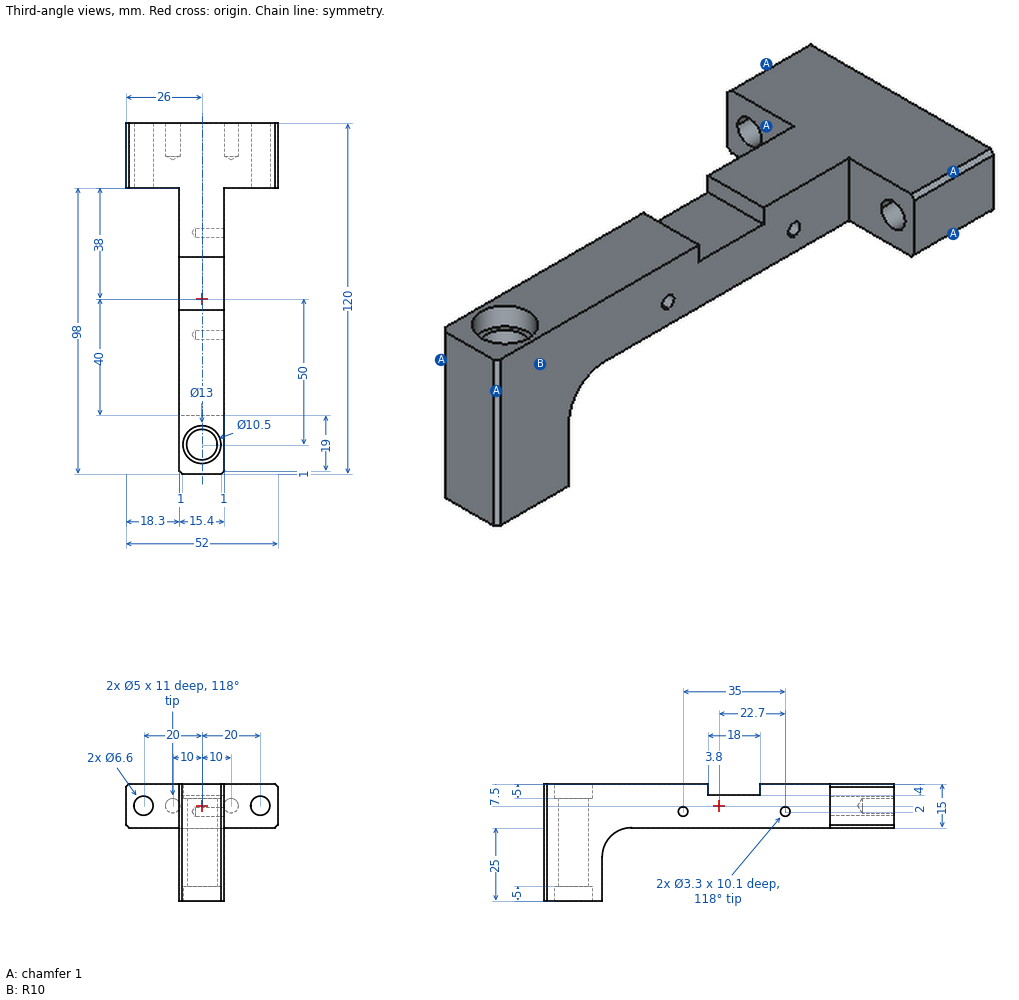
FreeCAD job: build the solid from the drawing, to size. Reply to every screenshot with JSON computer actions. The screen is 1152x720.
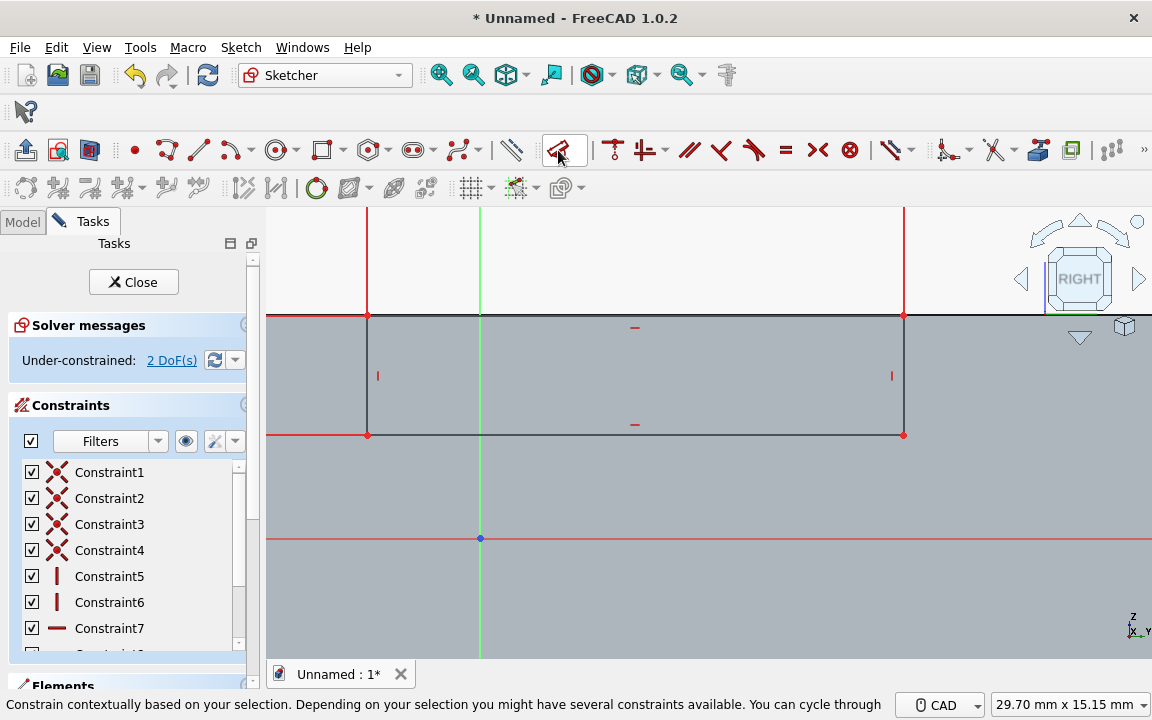
{"action": "left_click", "coordinate": [367, 316]}
{"action": "left_click", "coordinate": [424, 573]}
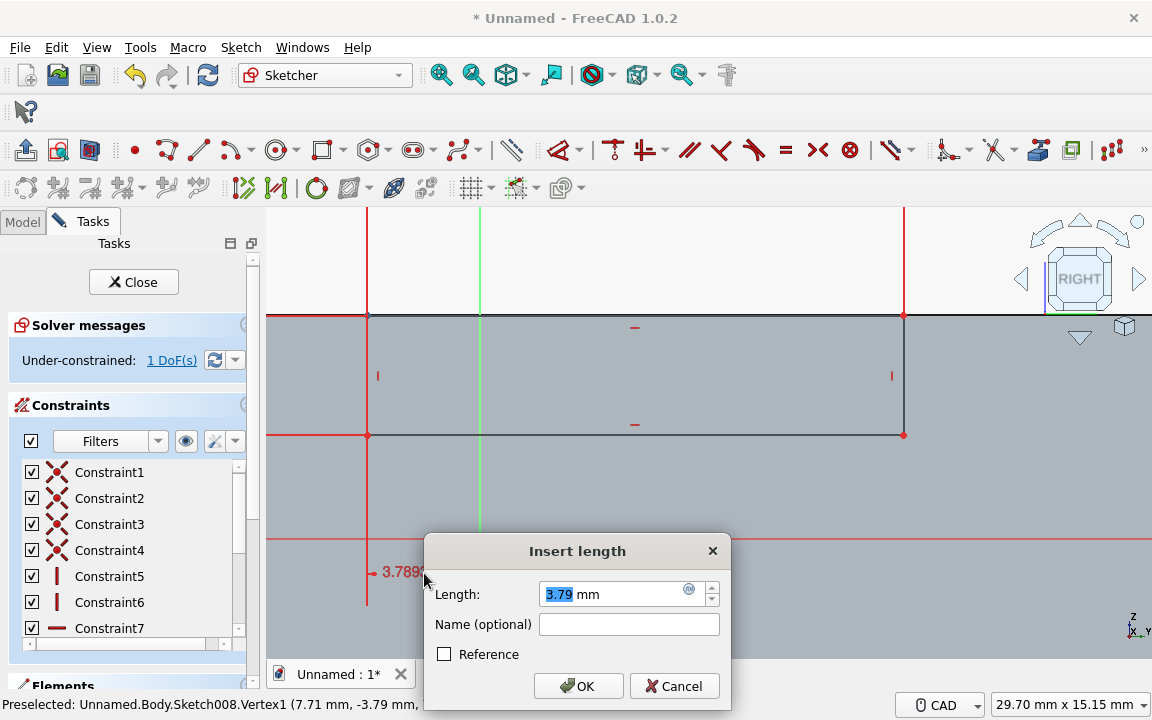
{"action": "type", "text": "3.8"}
{"action": "key", "text": "Return"}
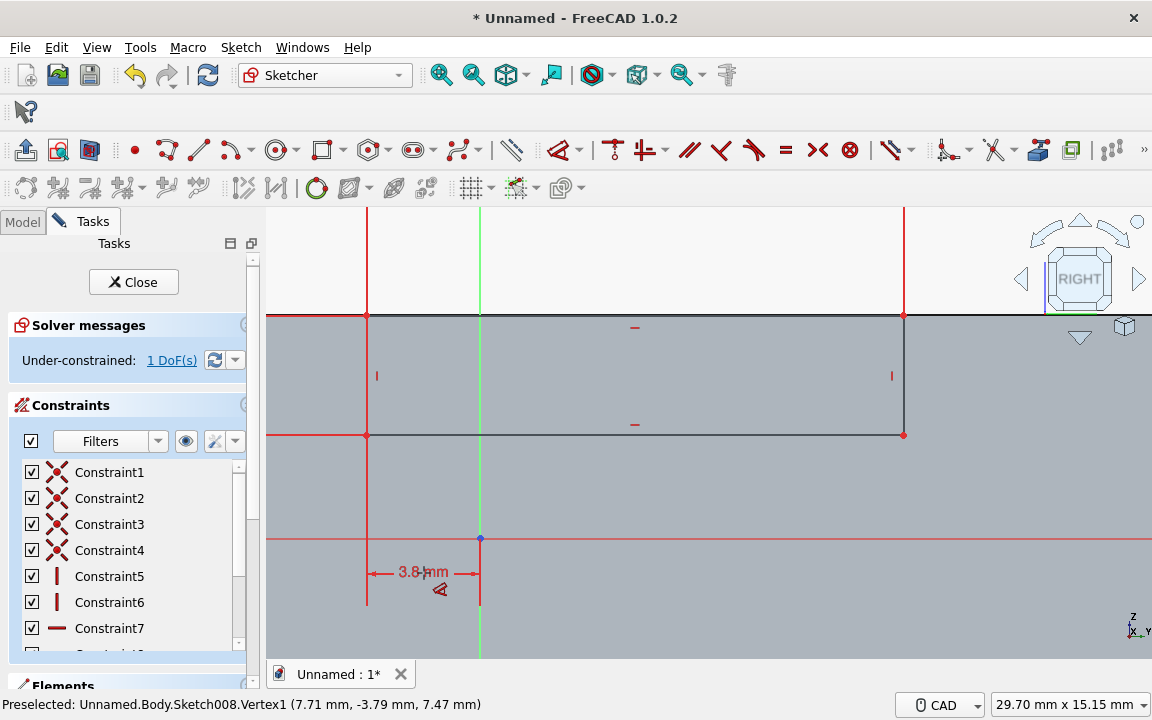
{"action": "left_click", "coordinate": [367, 316]}
{"action": "left_click", "coordinate": [333, 427]}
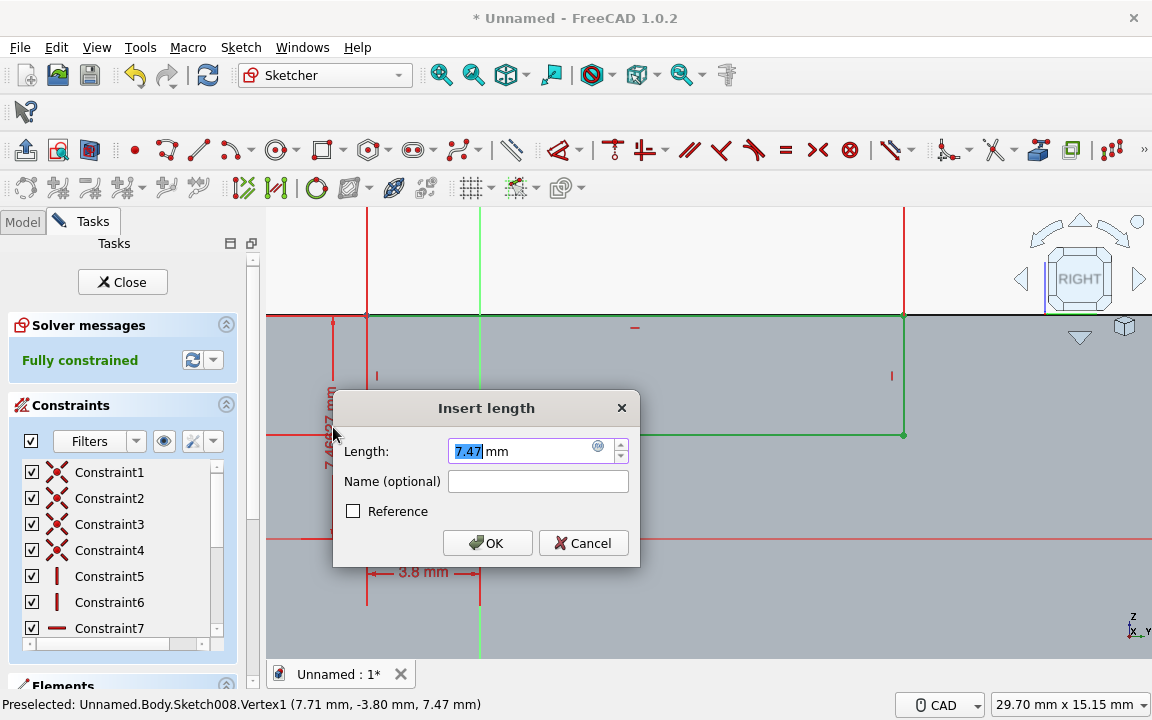
{"action": "type", "text": "7.5"}
{"action": "key", "text": "Return"}
{"action": "key", "text": "Escape"}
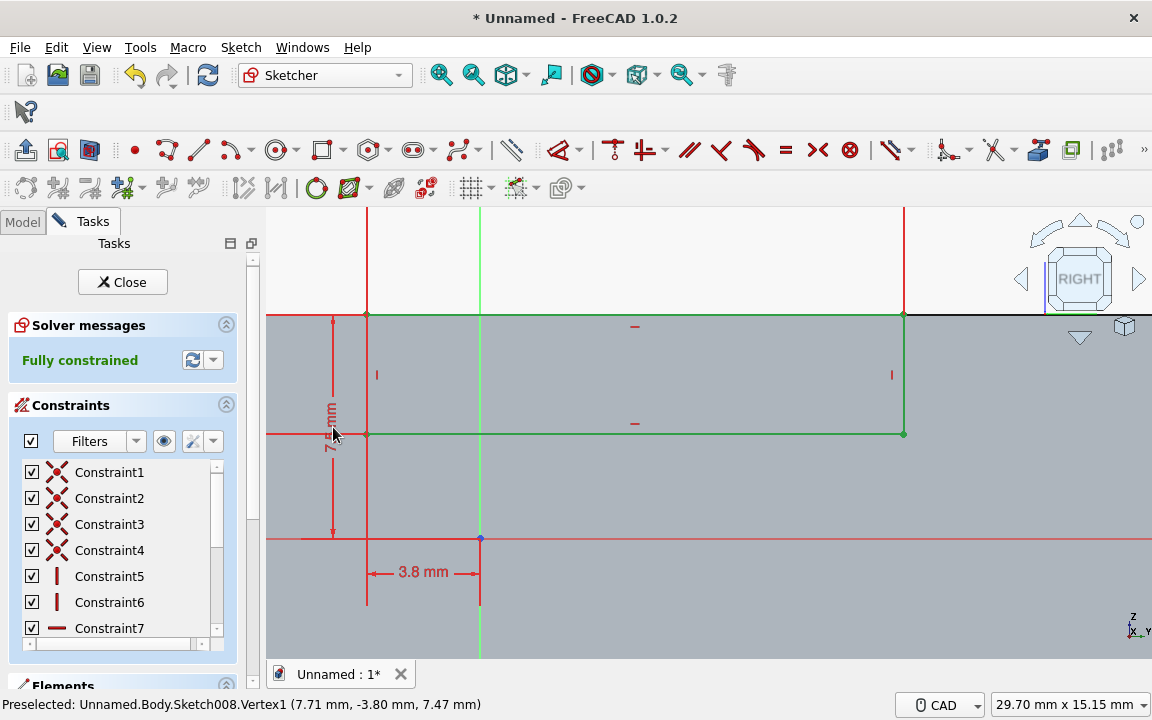
{"action": "left_click", "coordinate": [123, 282]}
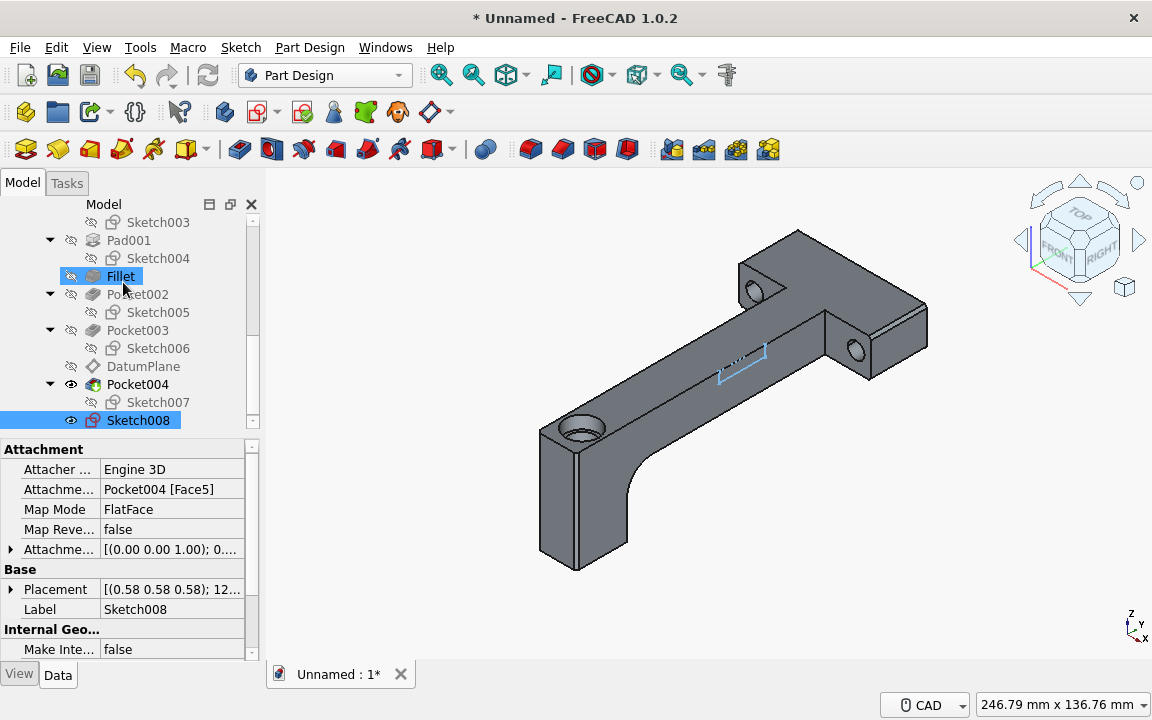
{"action": "left_click", "coordinate": [240, 150]}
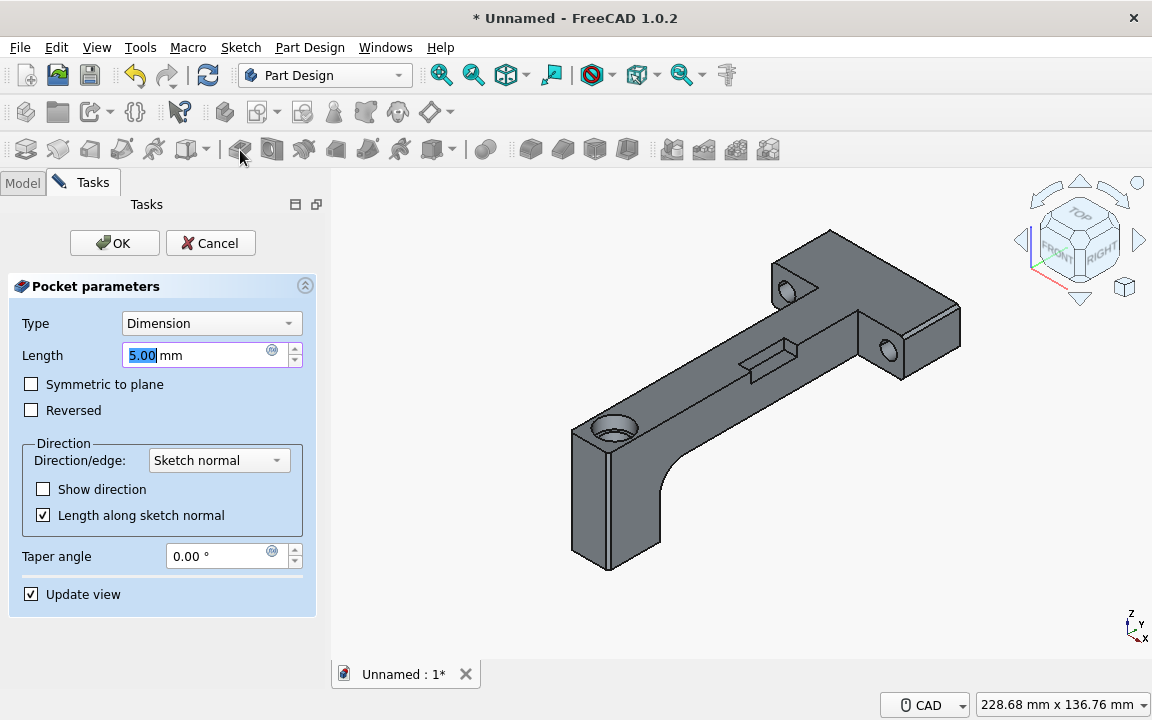
{"action": "left_click", "coordinate": [212, 324]}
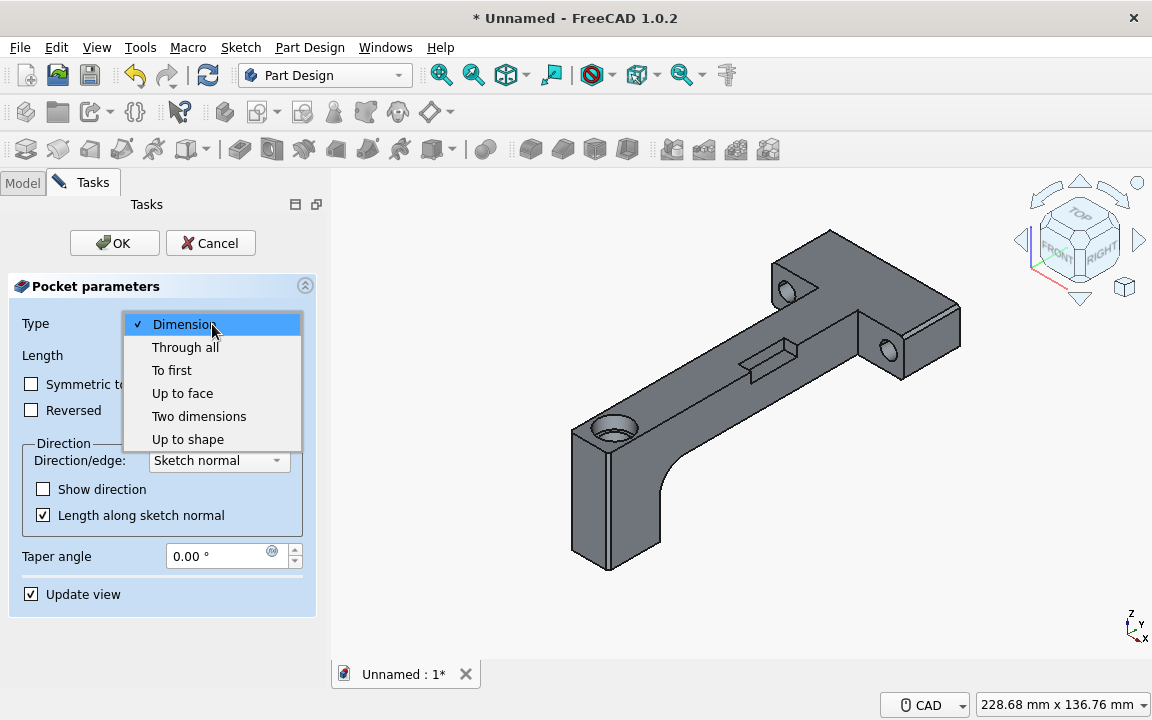
{"action": "left_click", "coordinate": [212, 348]}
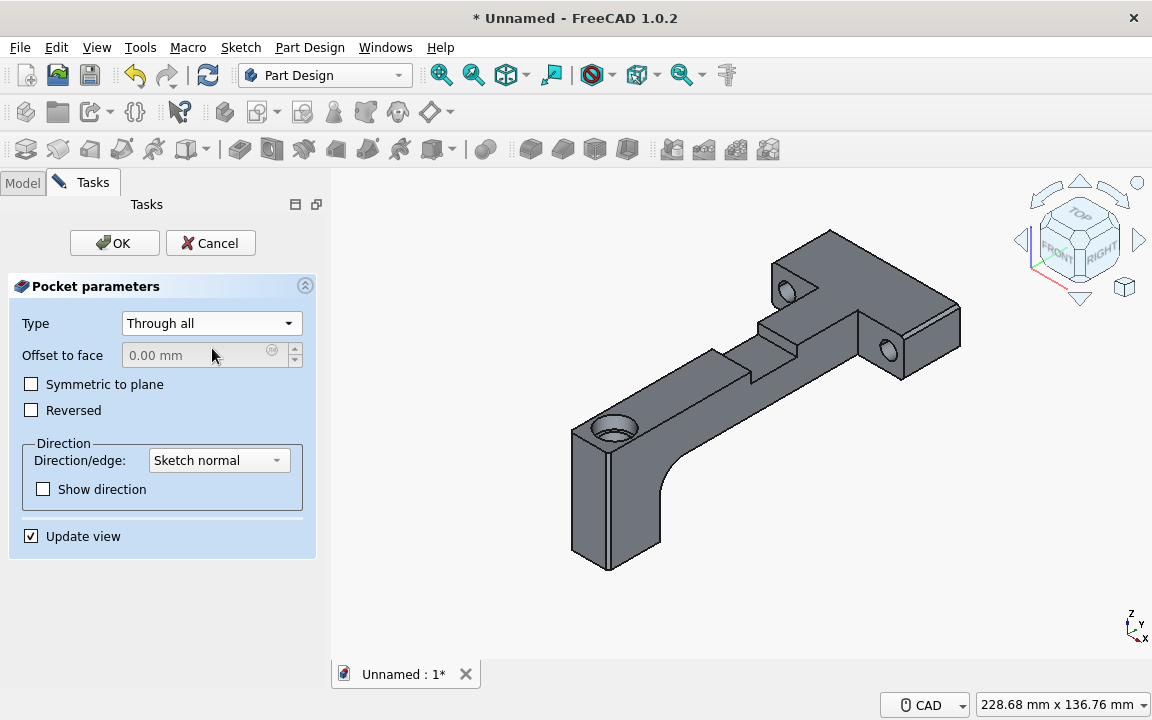
{"action": "left_click", "coordinate": [115, 243]}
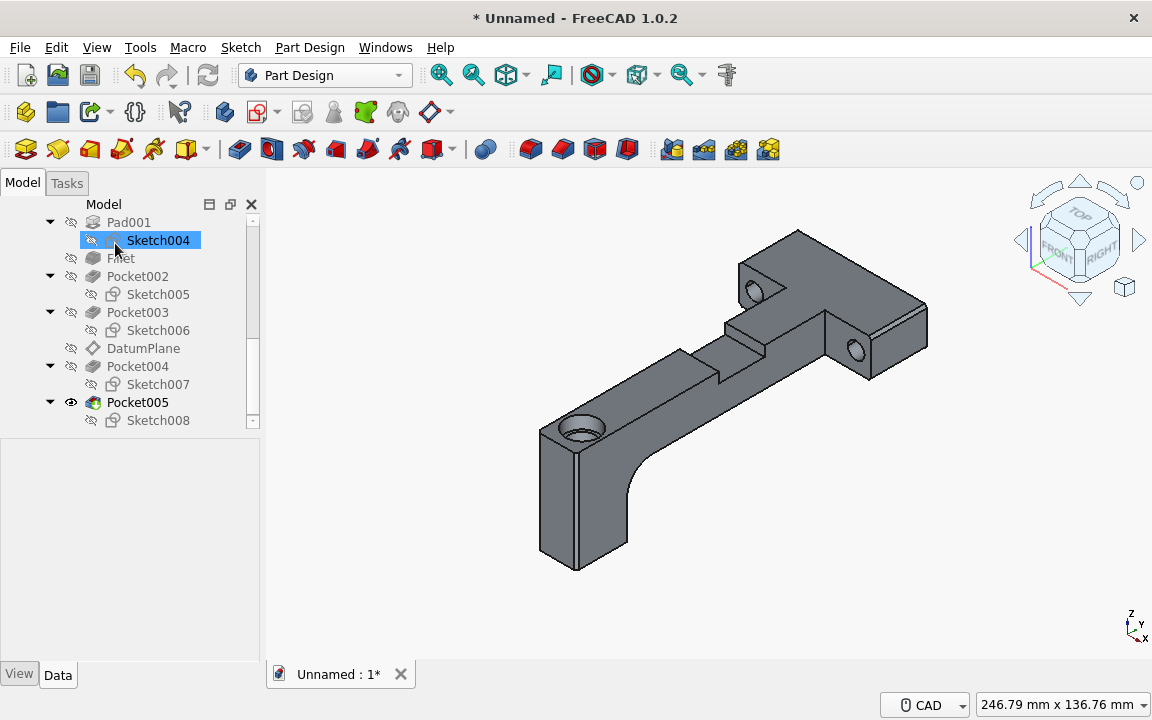
{"action": "left_click", "coordinate": [632, 446]}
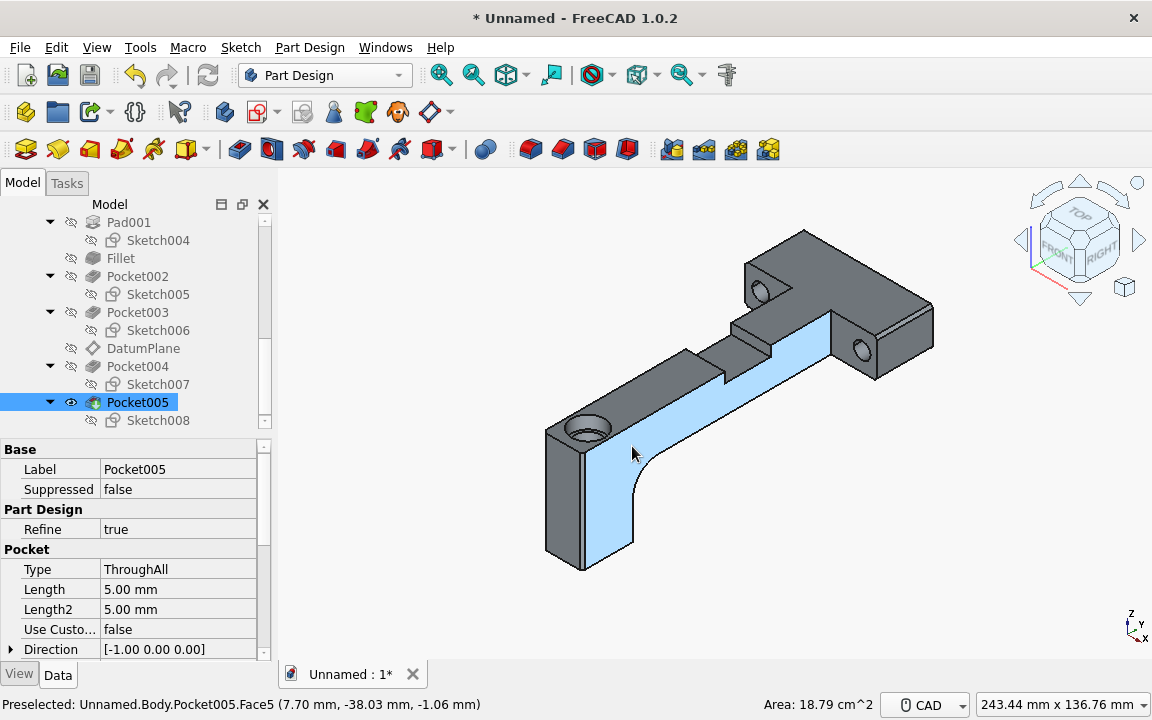
{"action": "left_click", "coordinate": [258, 112]}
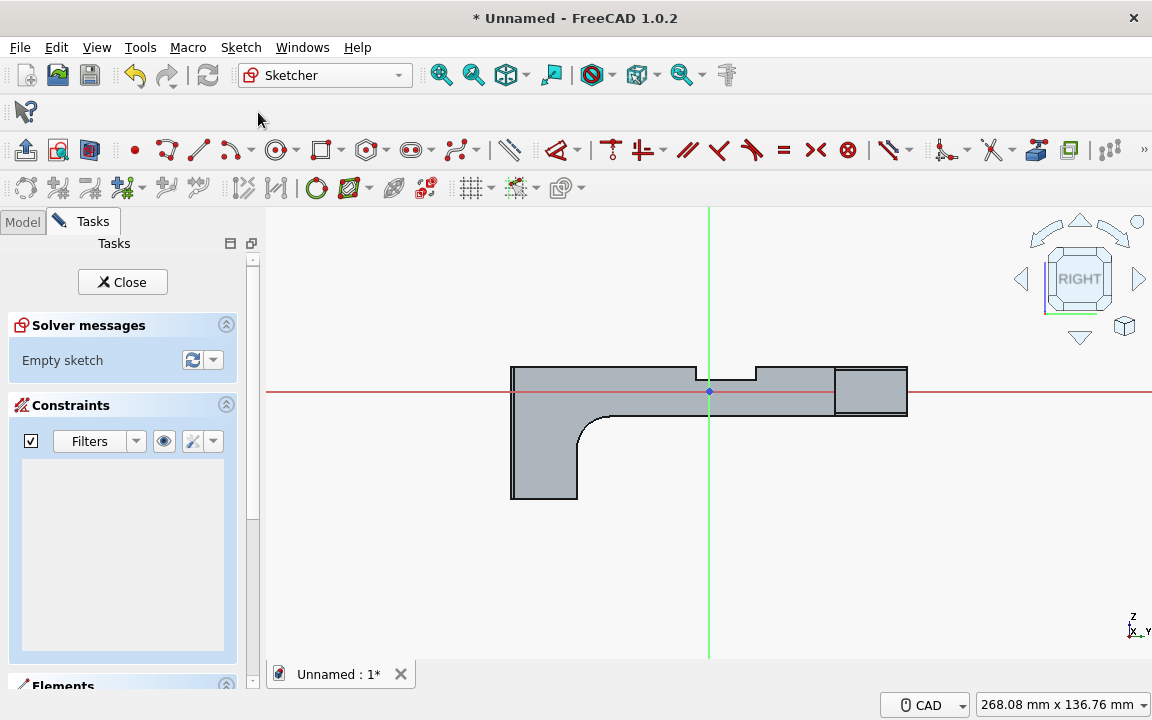
{"action": "scroll", "coordinate": [754, 386], "scroll_direction": "up", "scroll_amount": 7}